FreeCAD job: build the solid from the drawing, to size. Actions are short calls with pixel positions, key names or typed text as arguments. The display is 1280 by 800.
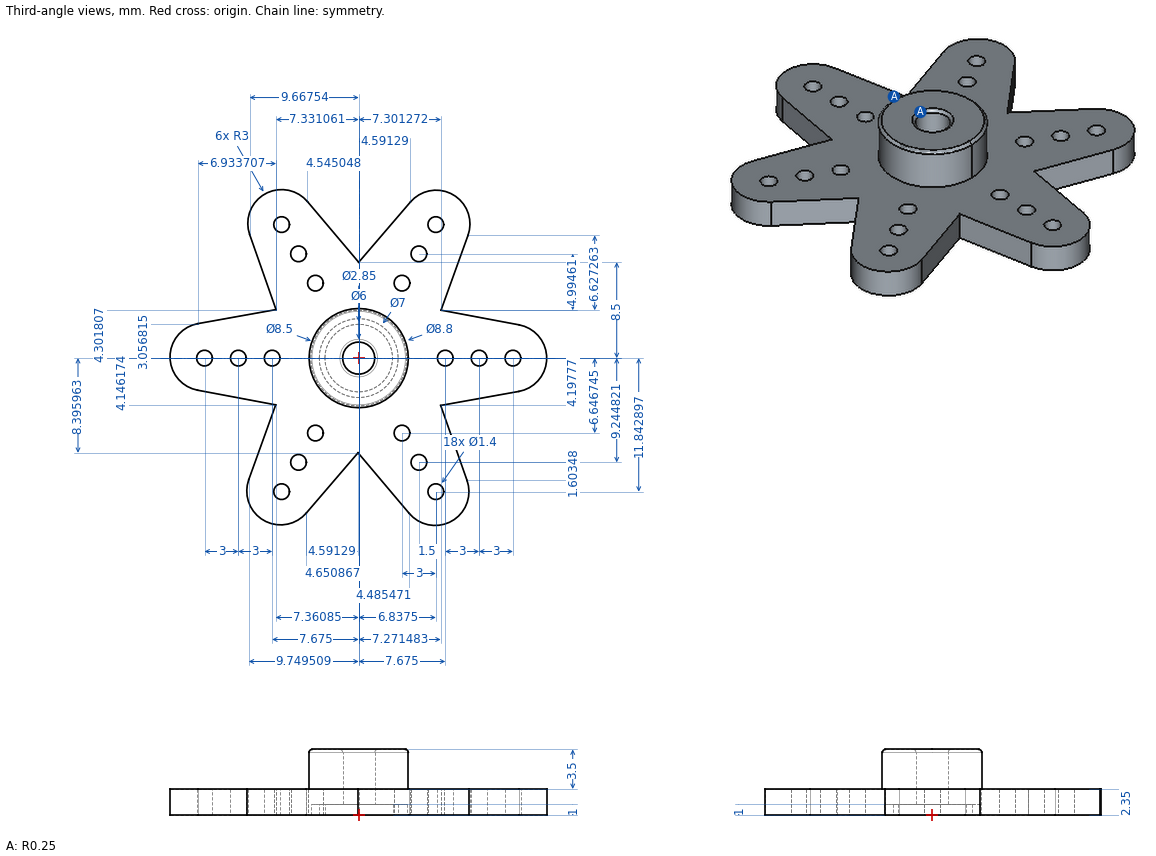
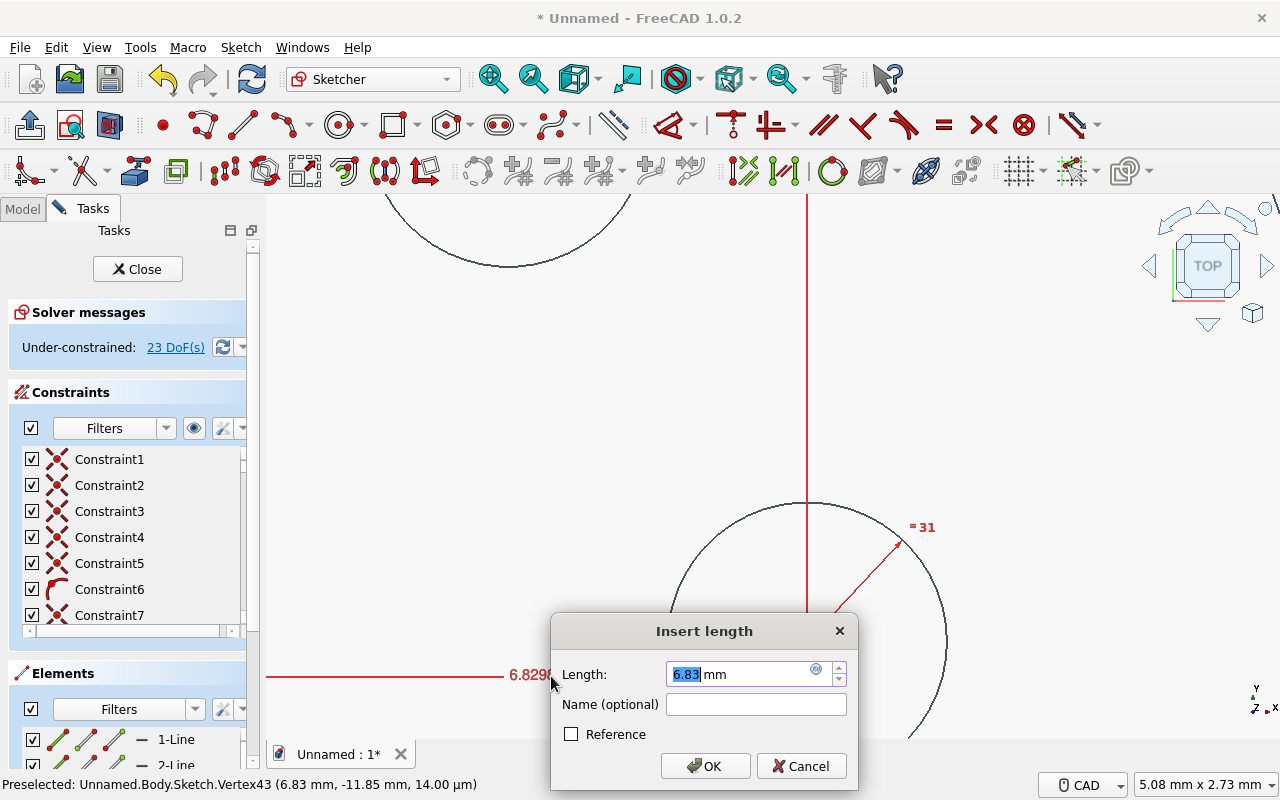
text(6.8375)
key(Return)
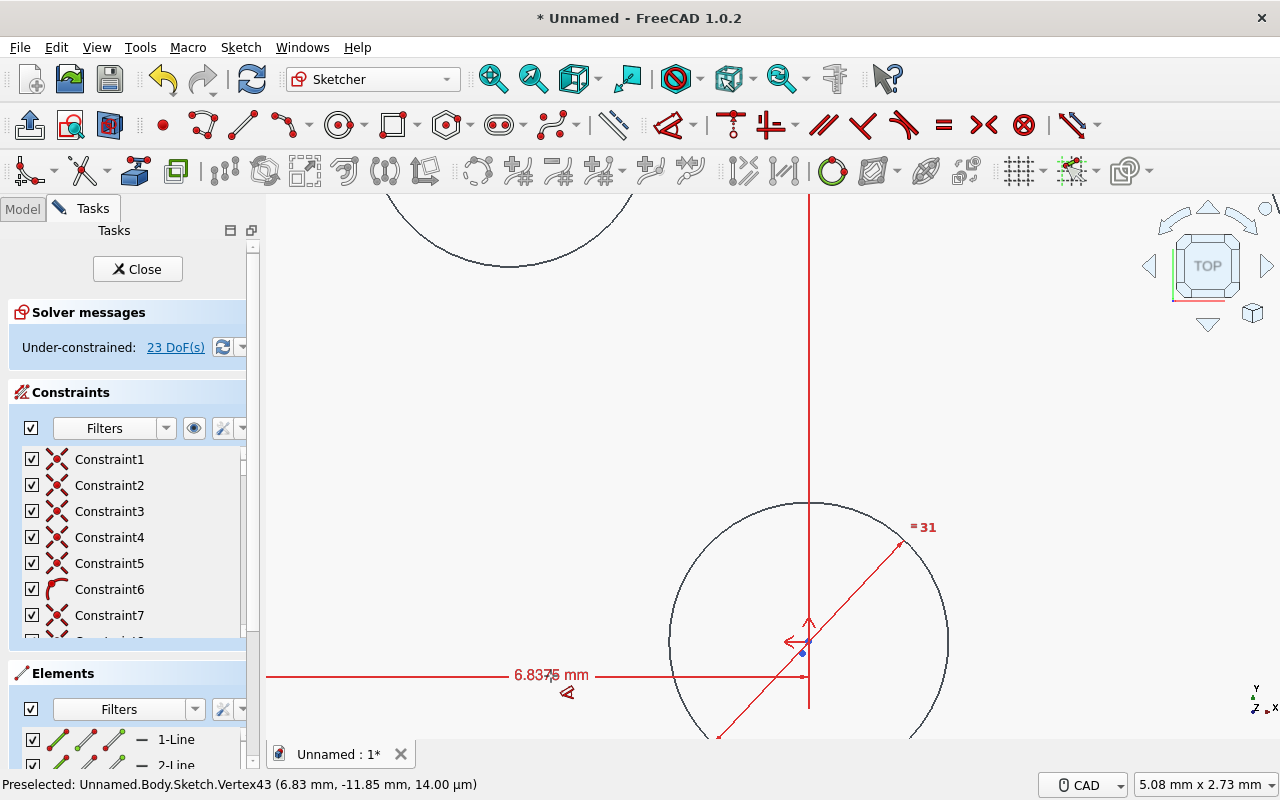
scroll(786, 609, down, 14)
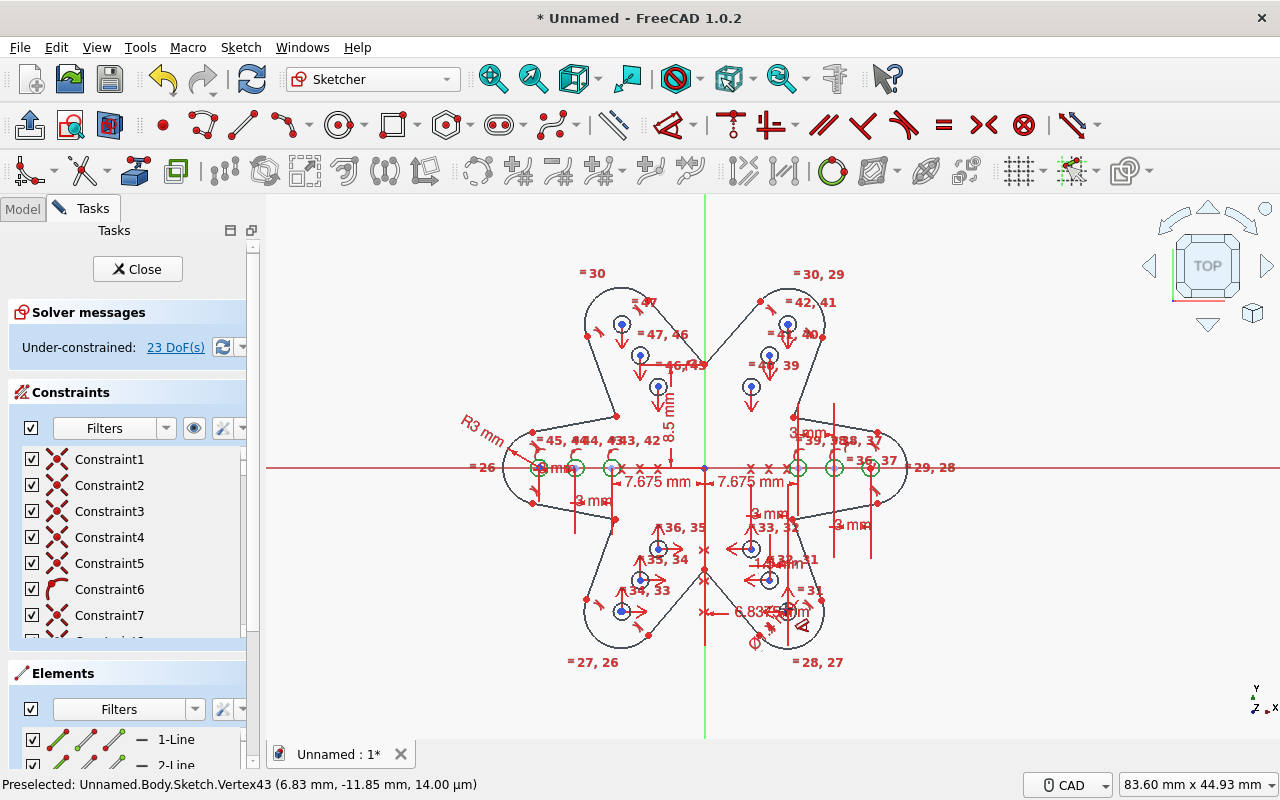
click(587, 337)
click(619, 303)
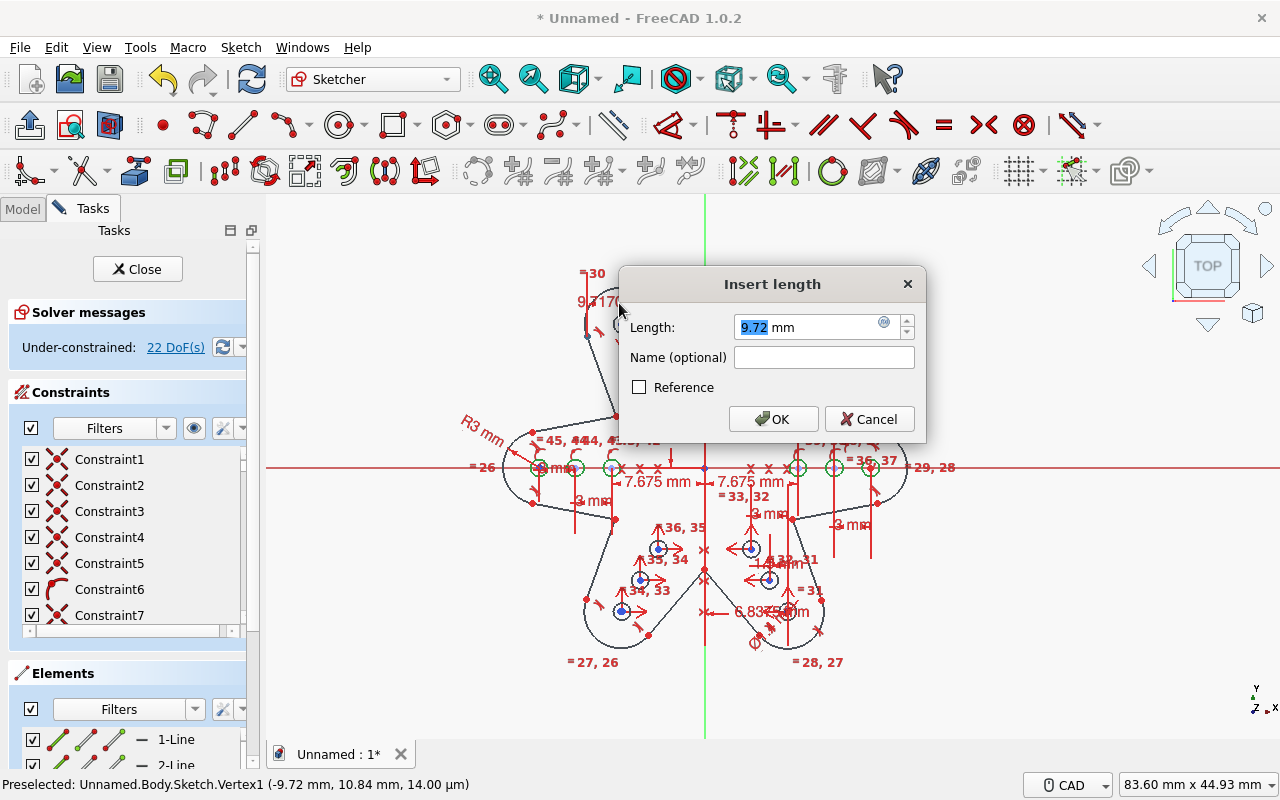
text(9.66754)
key(Return)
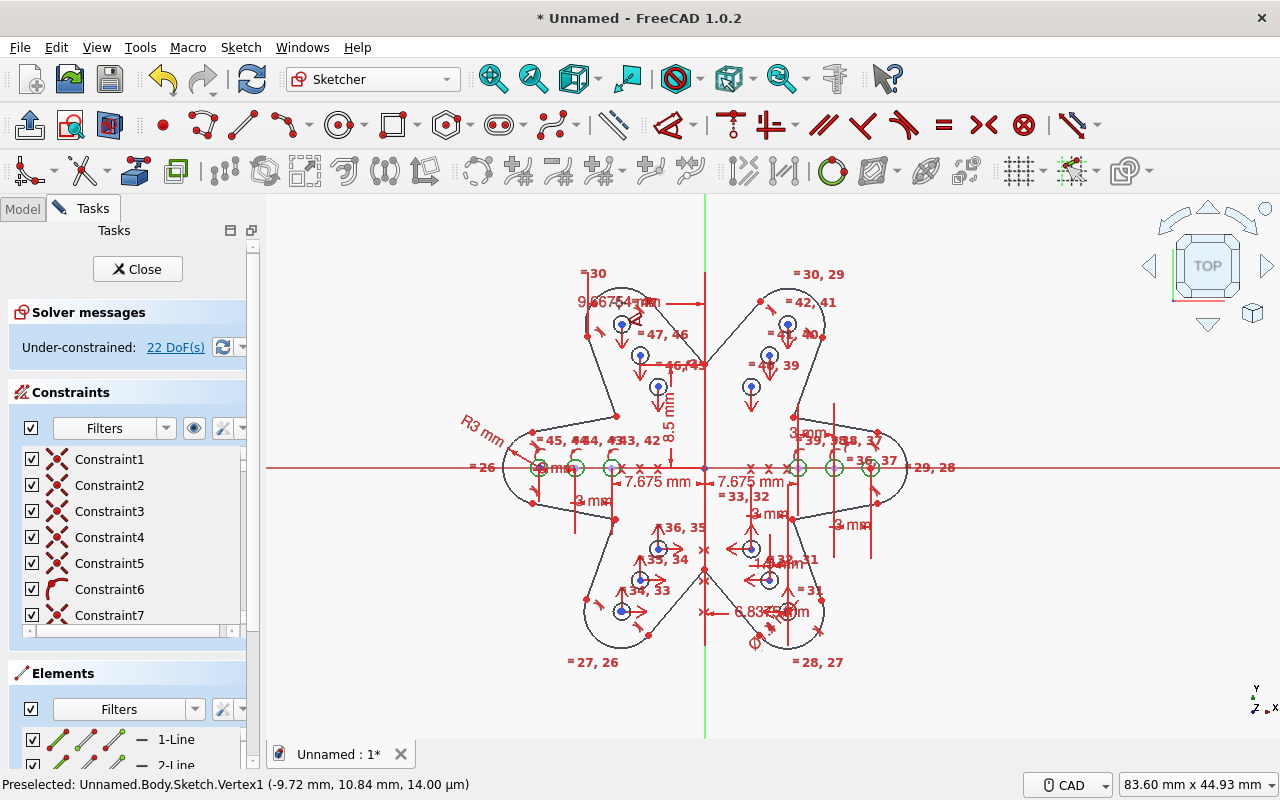
click(615, 520)
click(681, 554)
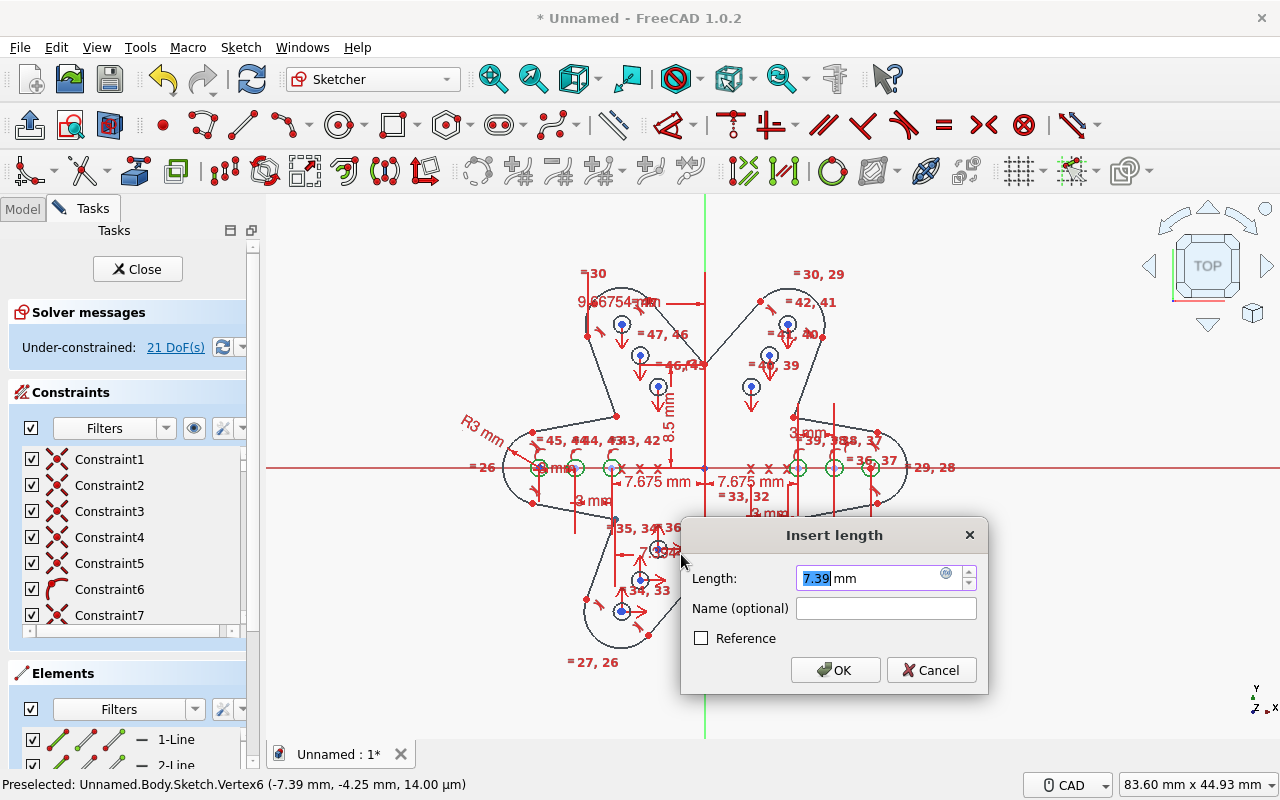
text(7.36085)
key(Return)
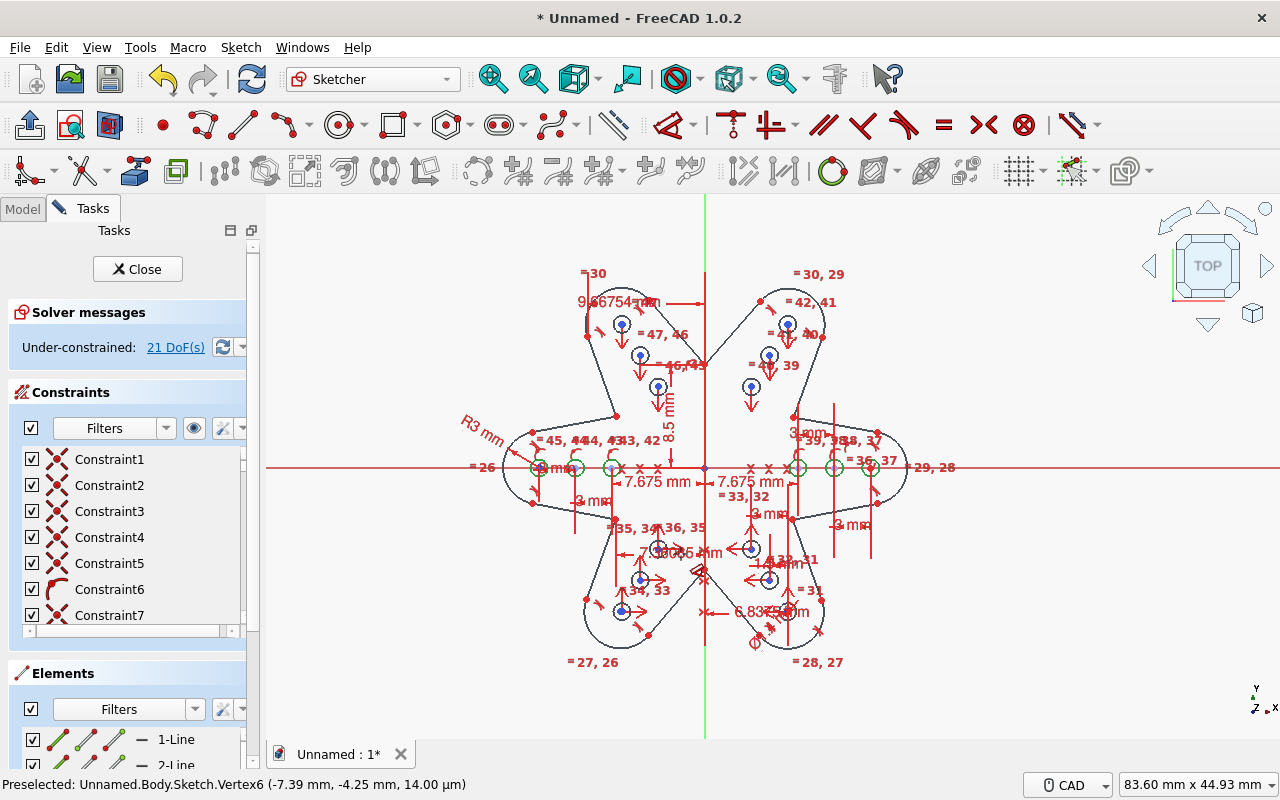
click(793, 520)
click(827, 494)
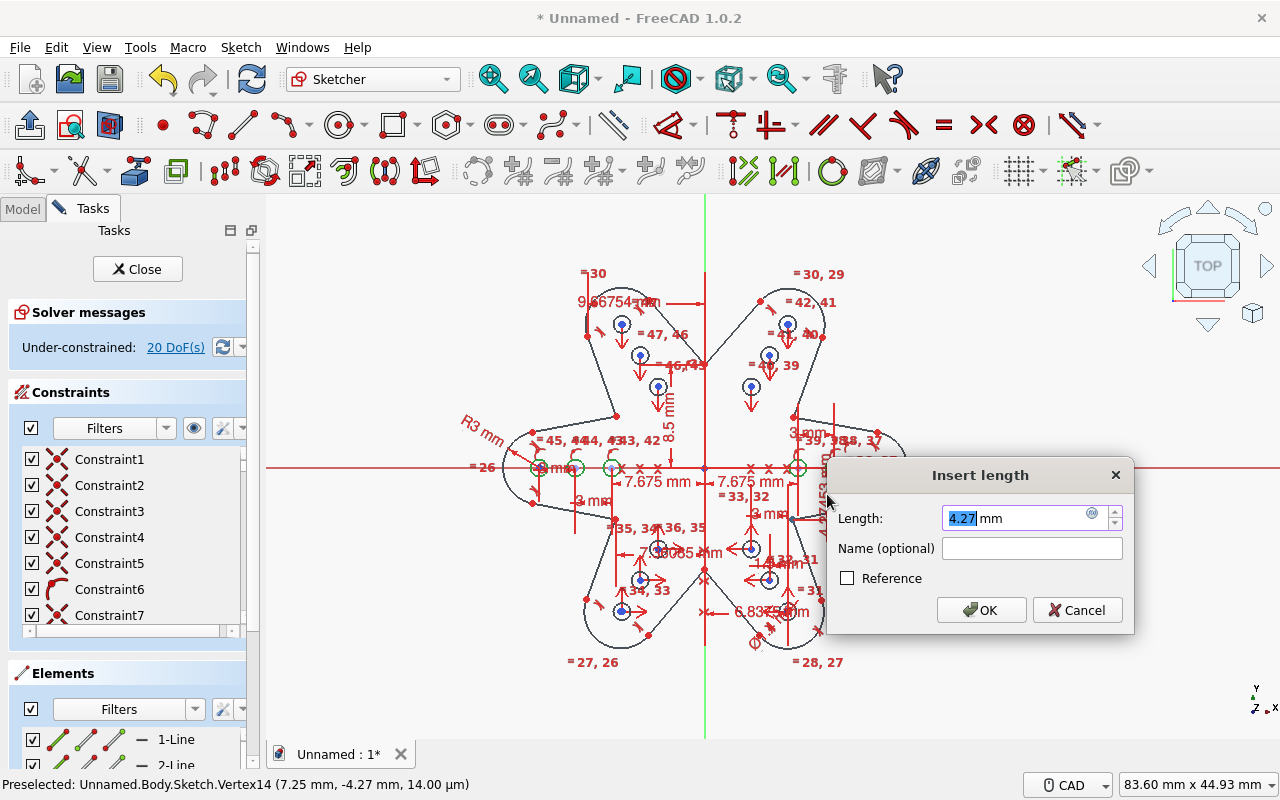
text(4.19777)
key(Return)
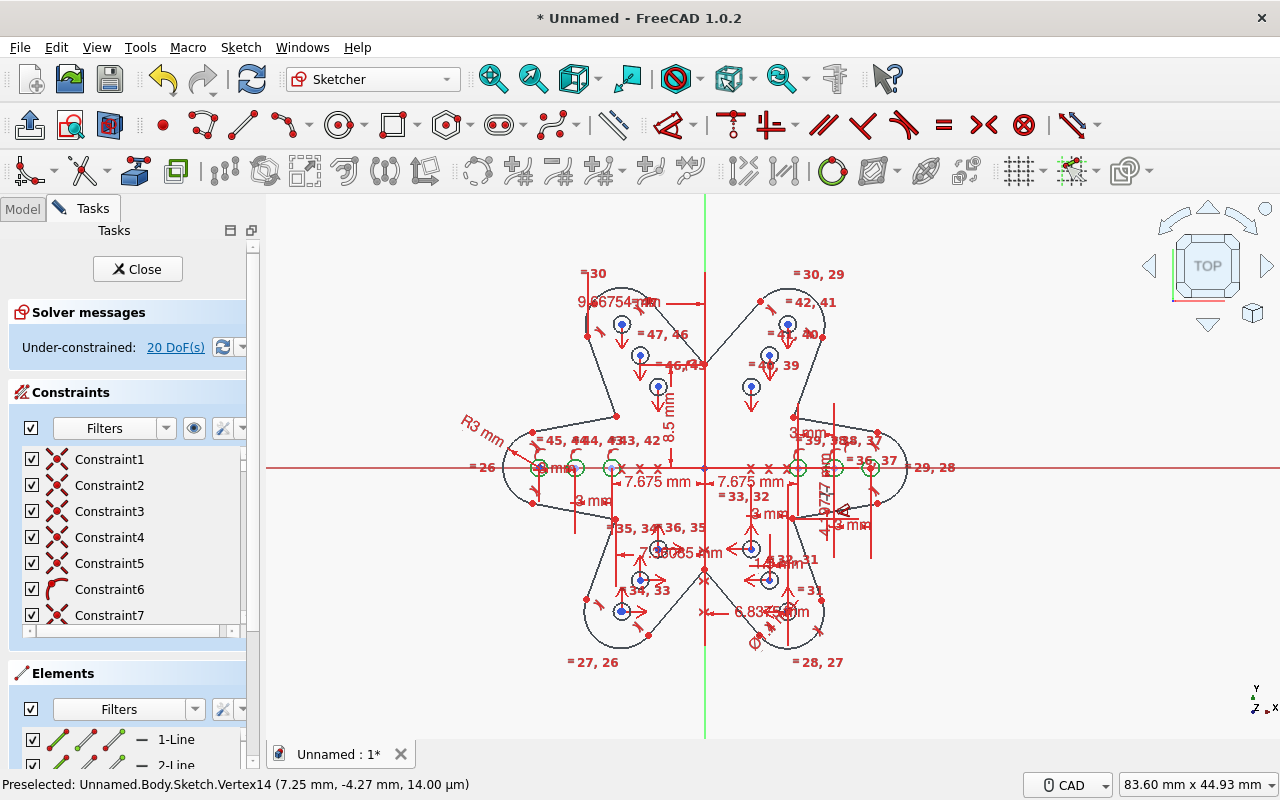
click(761, 301)
click(733, 267)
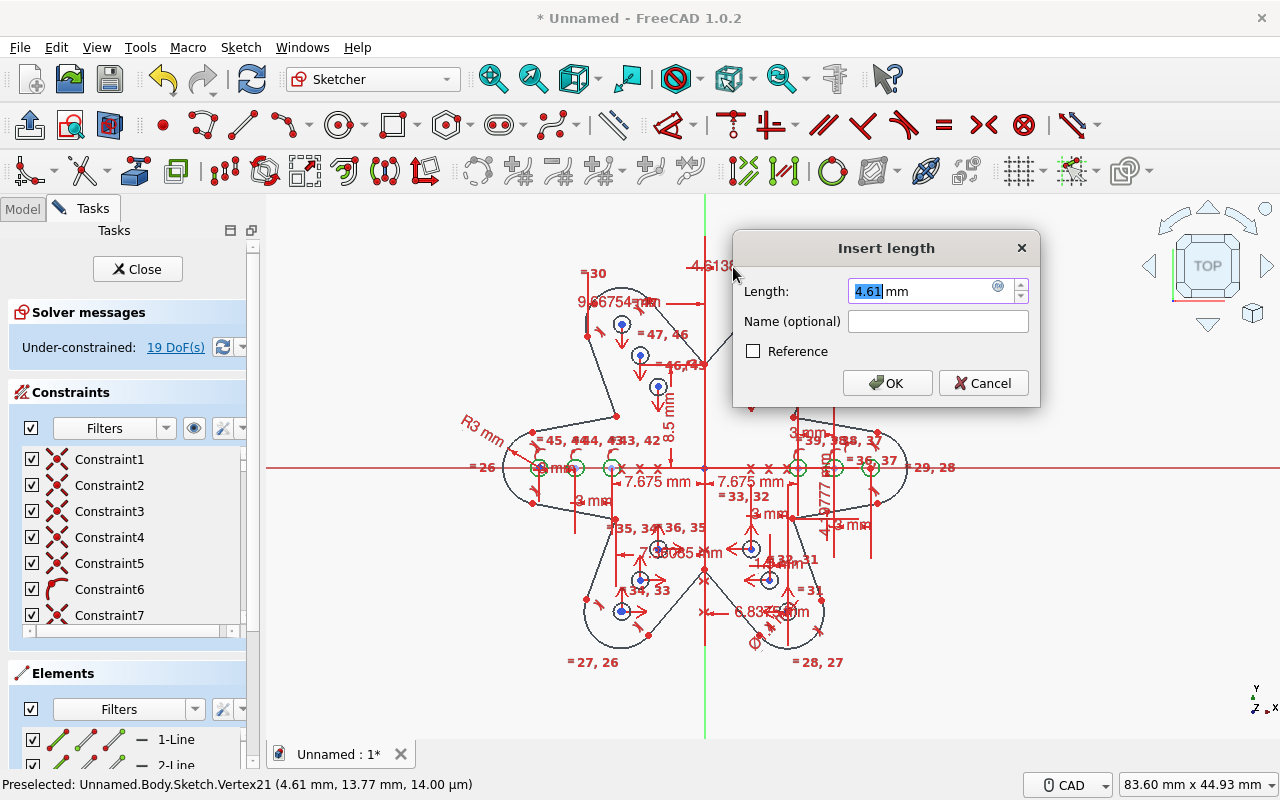
text(4.59129)
key(Return)